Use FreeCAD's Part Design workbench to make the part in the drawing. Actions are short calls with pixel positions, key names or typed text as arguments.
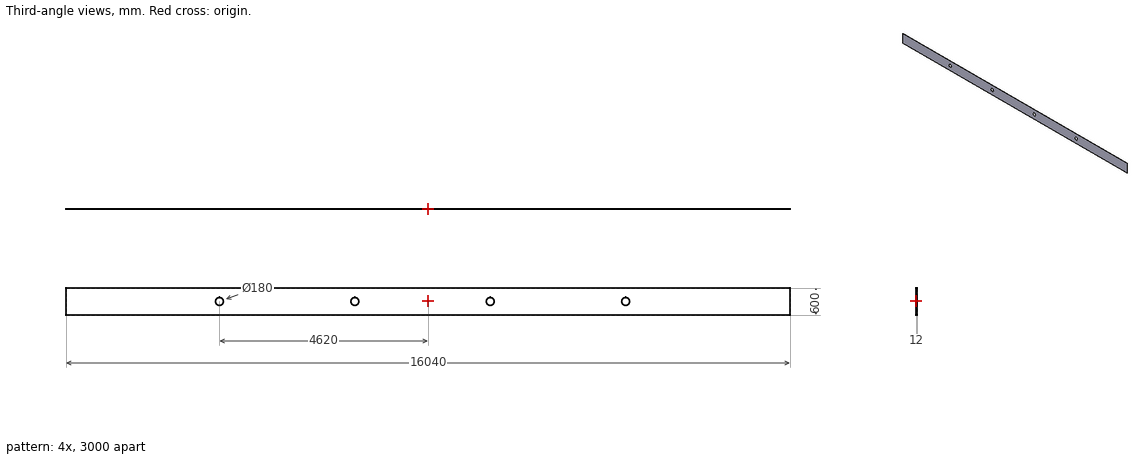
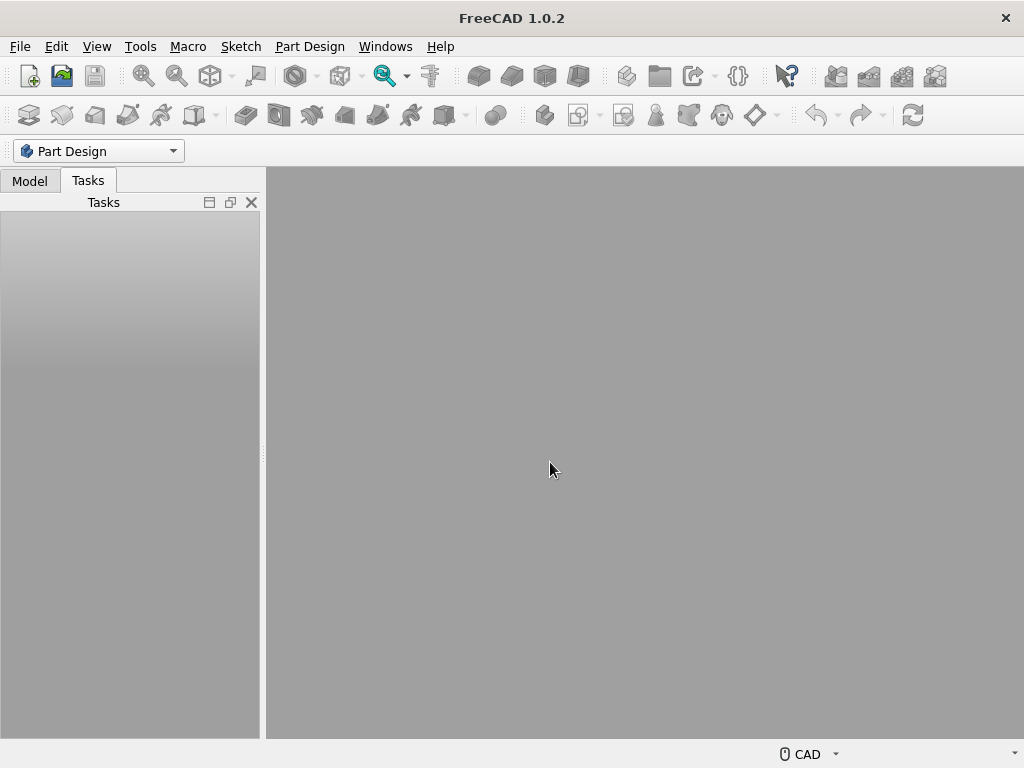
click(29, 76)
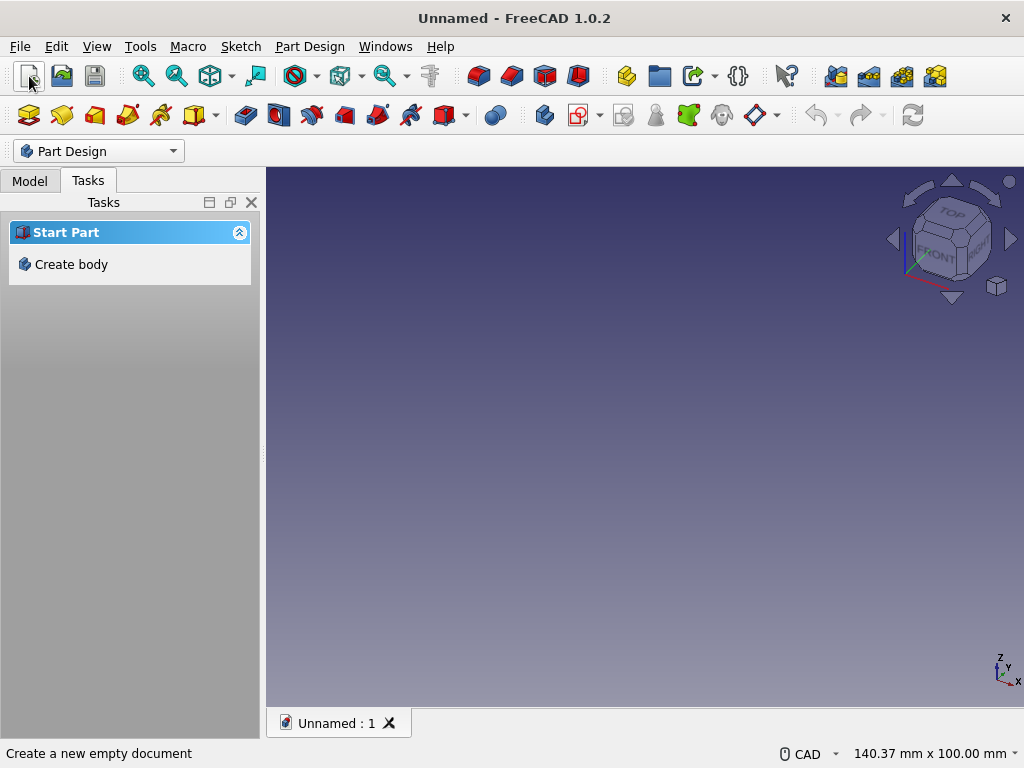
click(578, 116)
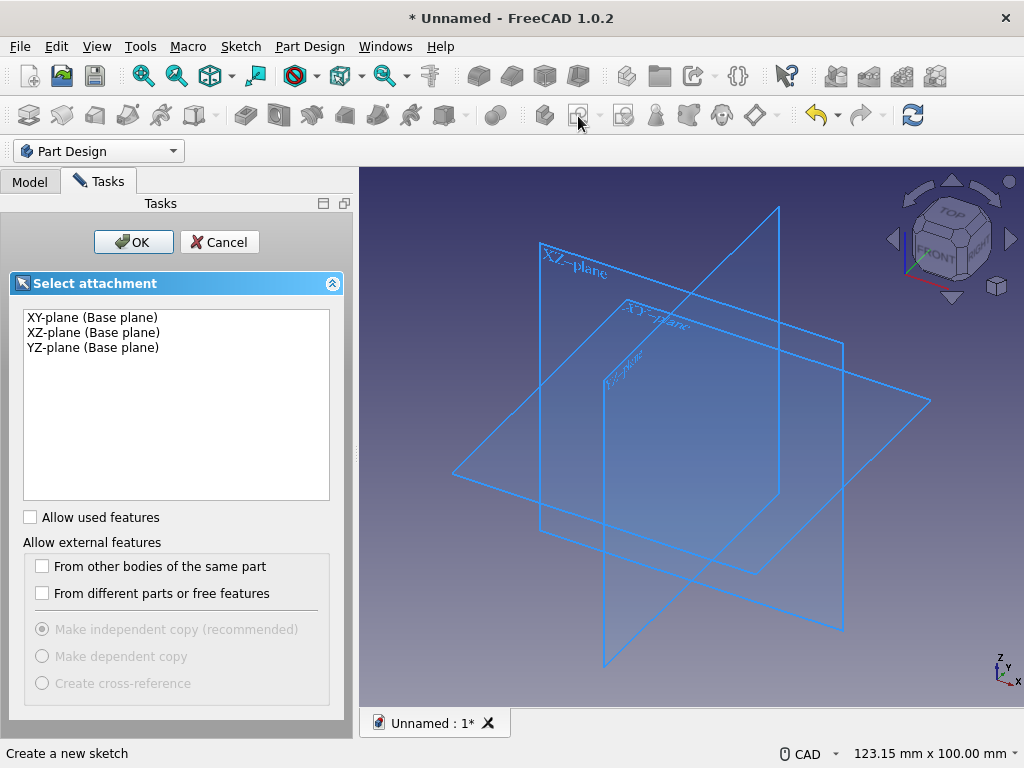
click(84, 332)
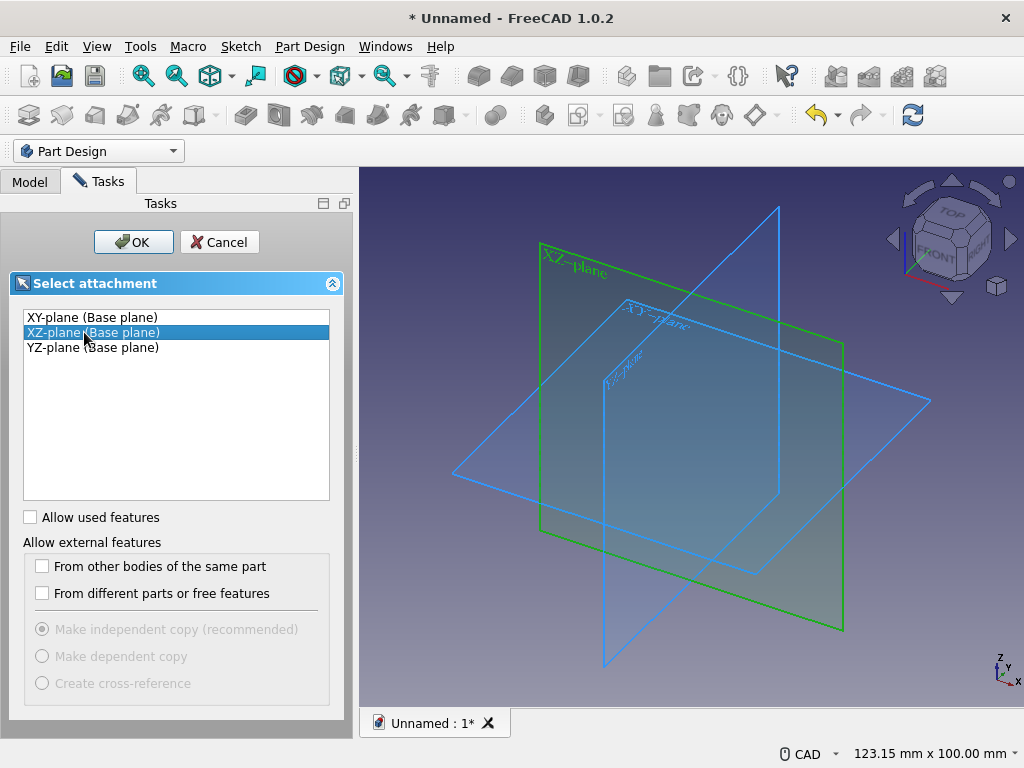
click(134, 242)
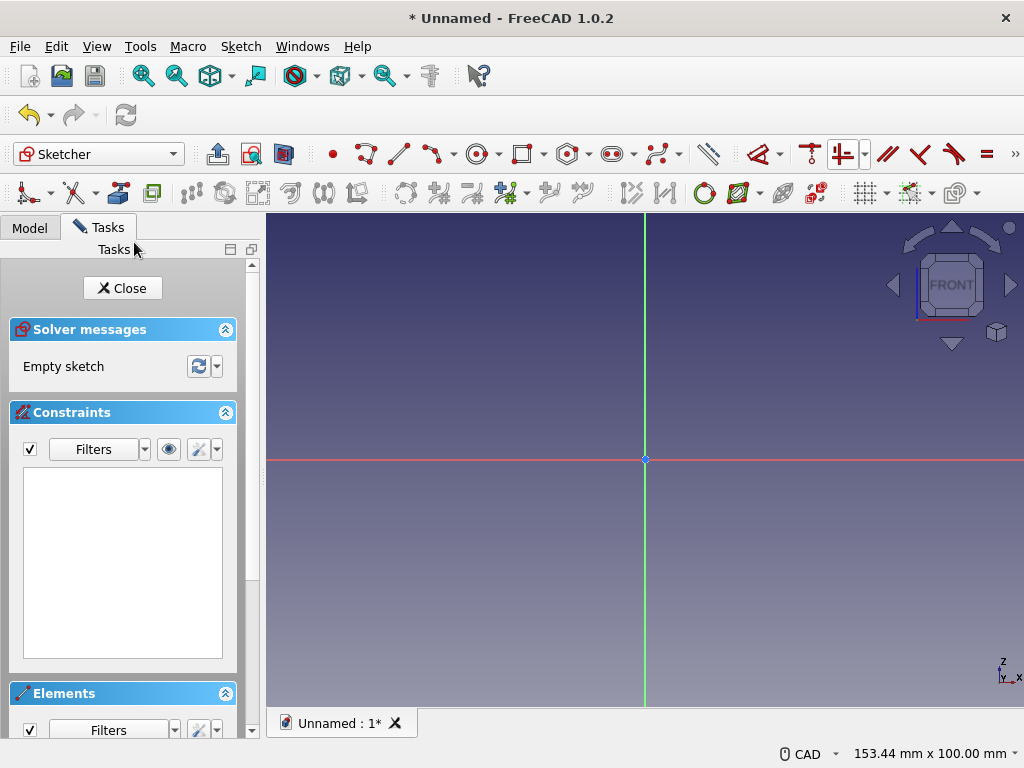
scroll(576, 460, down, 15)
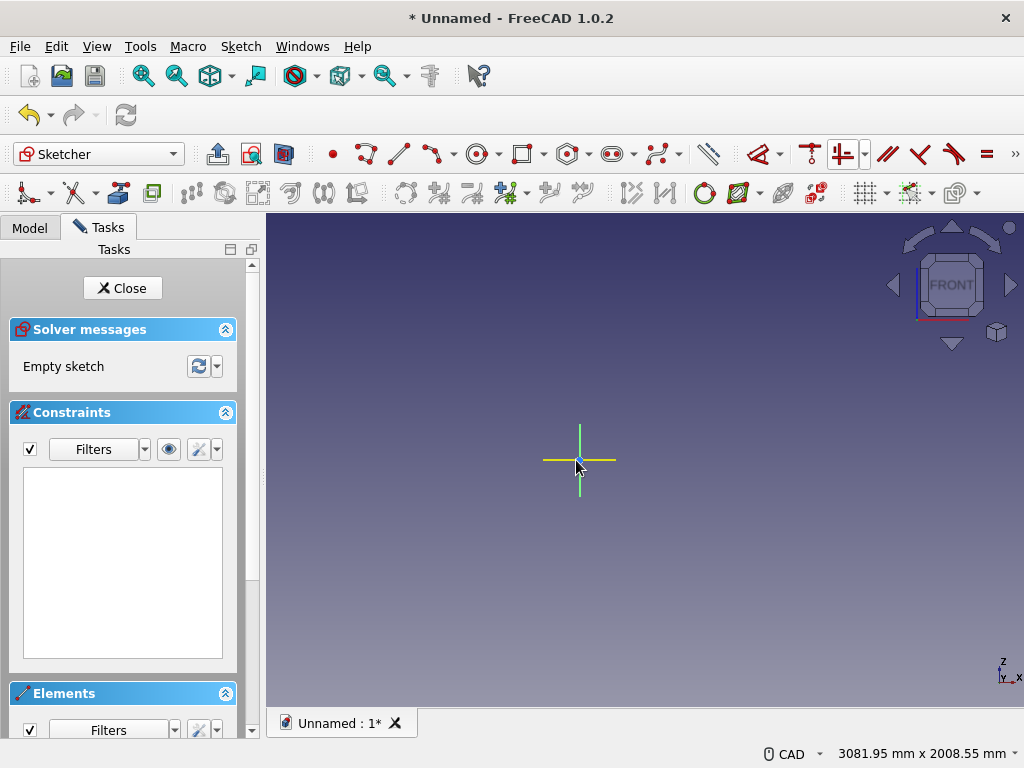
scroll(576, 460, down, 11)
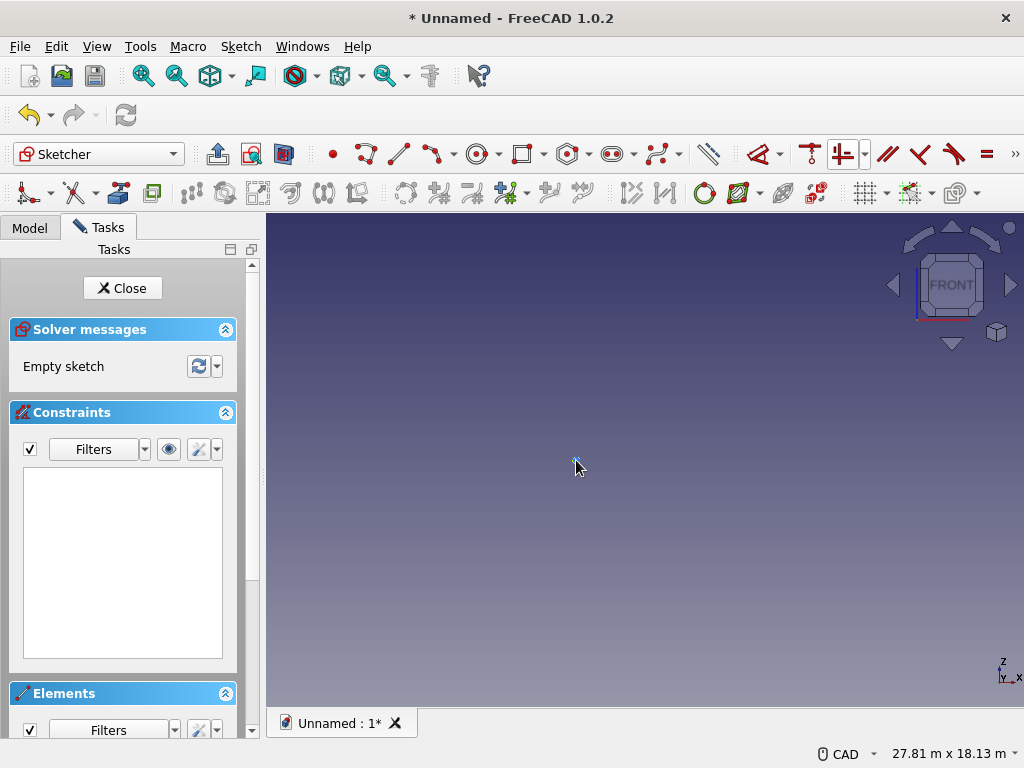
click(544, 154)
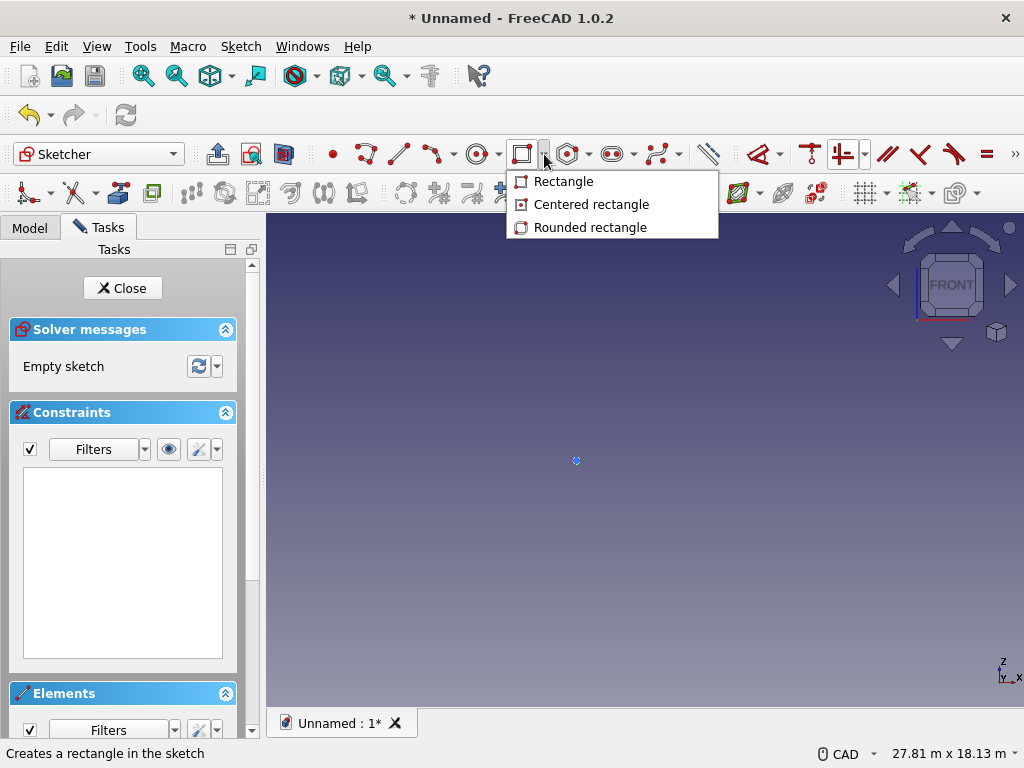
click(612, 204)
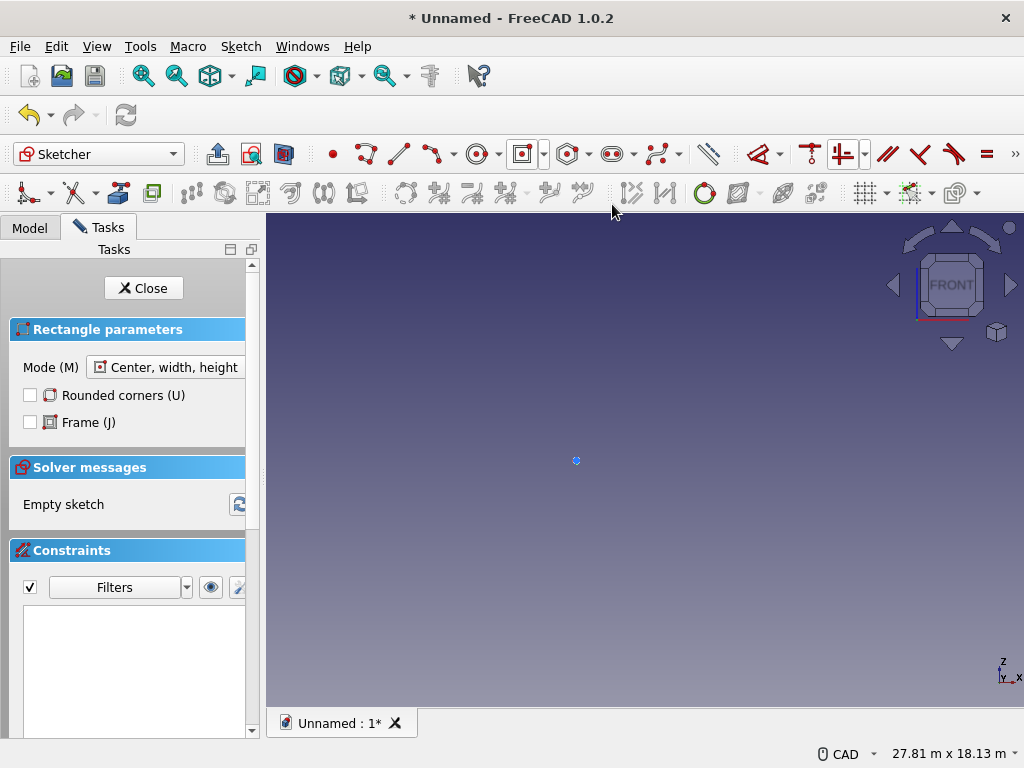
scroll(577, 460, up, 4)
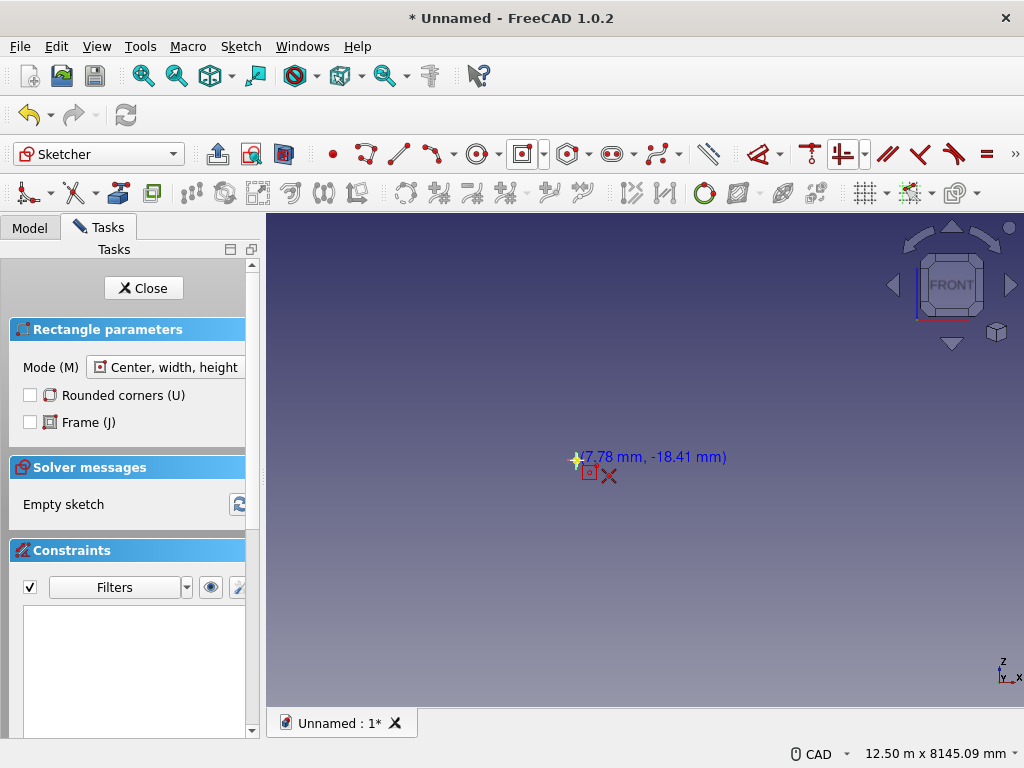
click(576, 460)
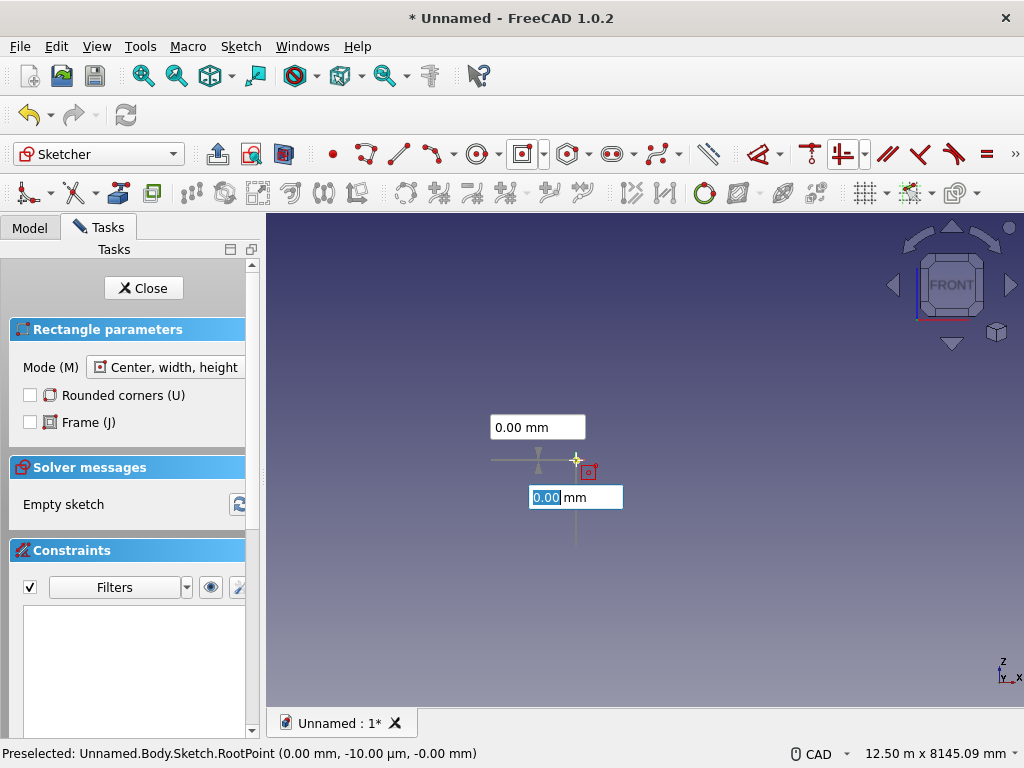
scroll(577, 460, down, 4)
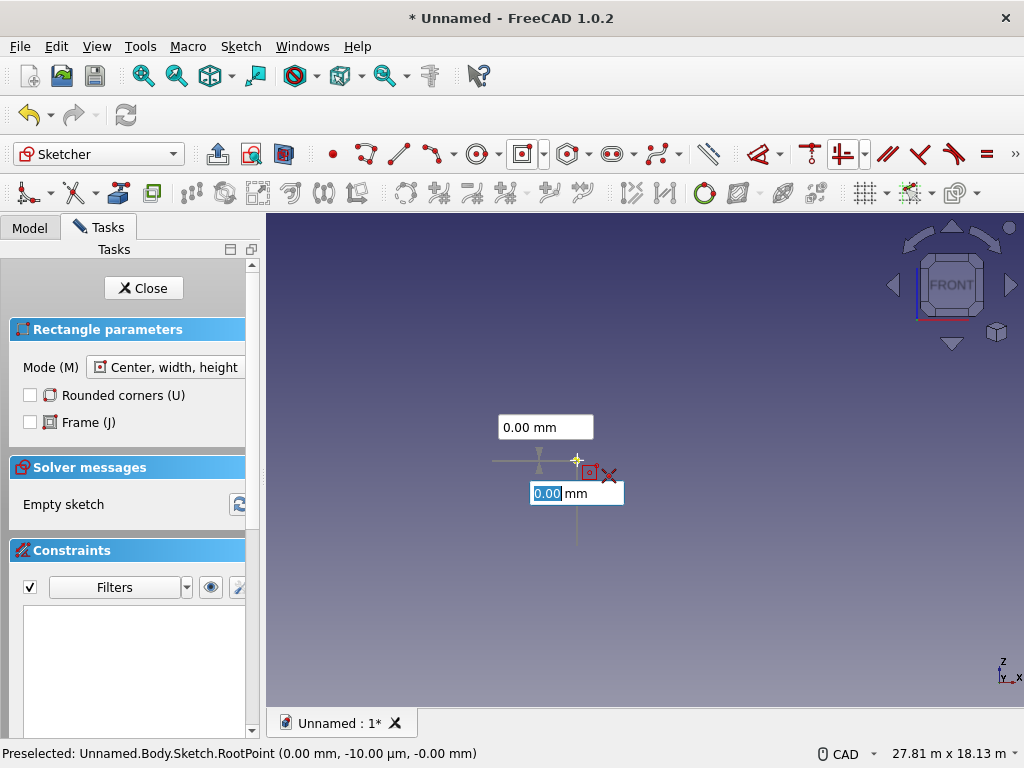
scroll(795, 452, up, 4)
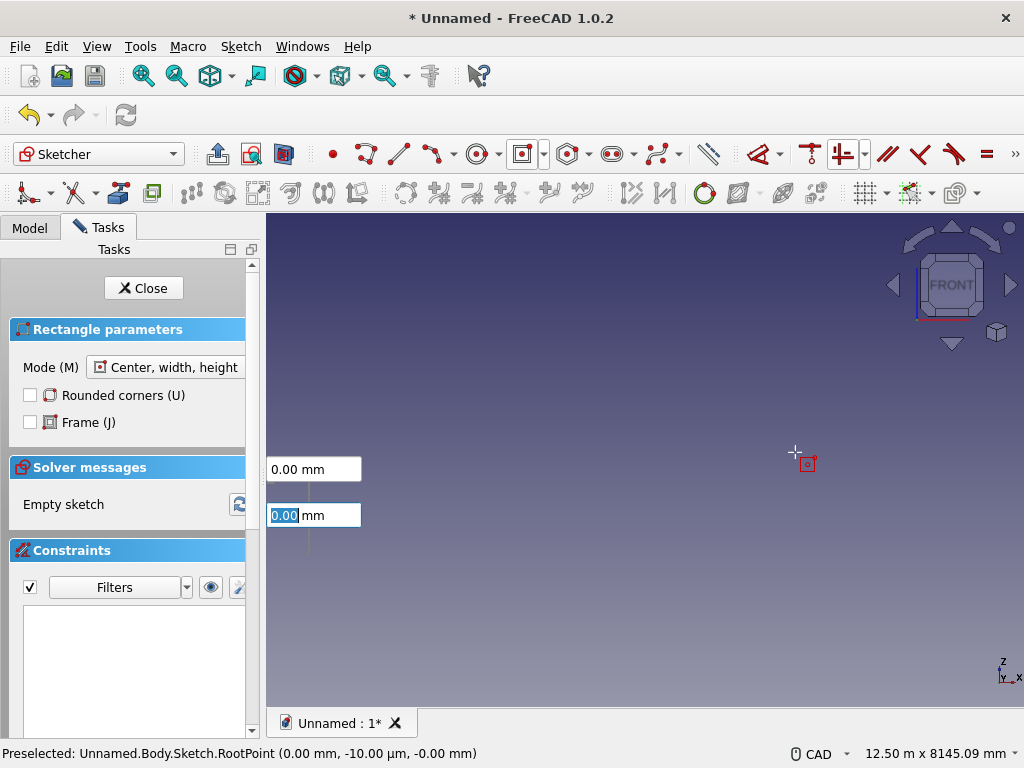
click(795, 452)
key(Escape)